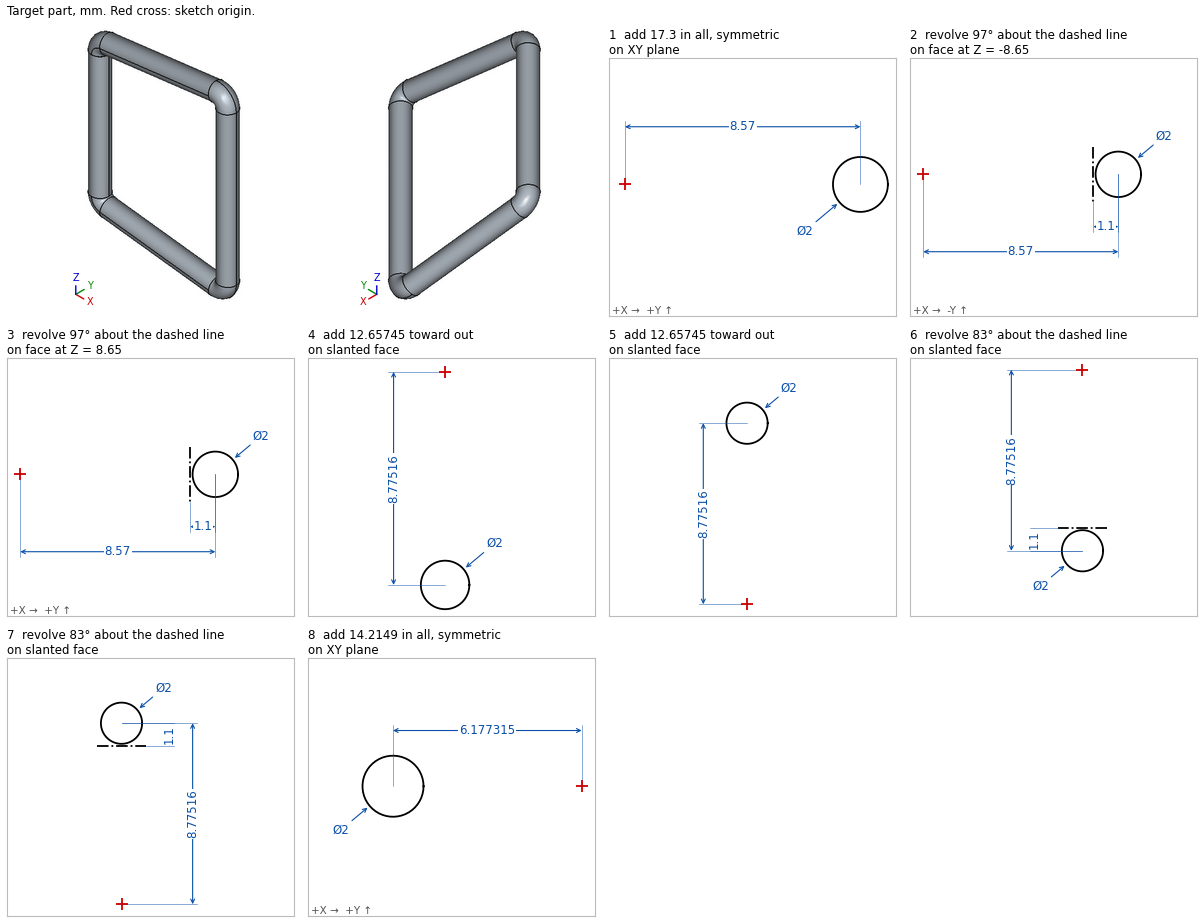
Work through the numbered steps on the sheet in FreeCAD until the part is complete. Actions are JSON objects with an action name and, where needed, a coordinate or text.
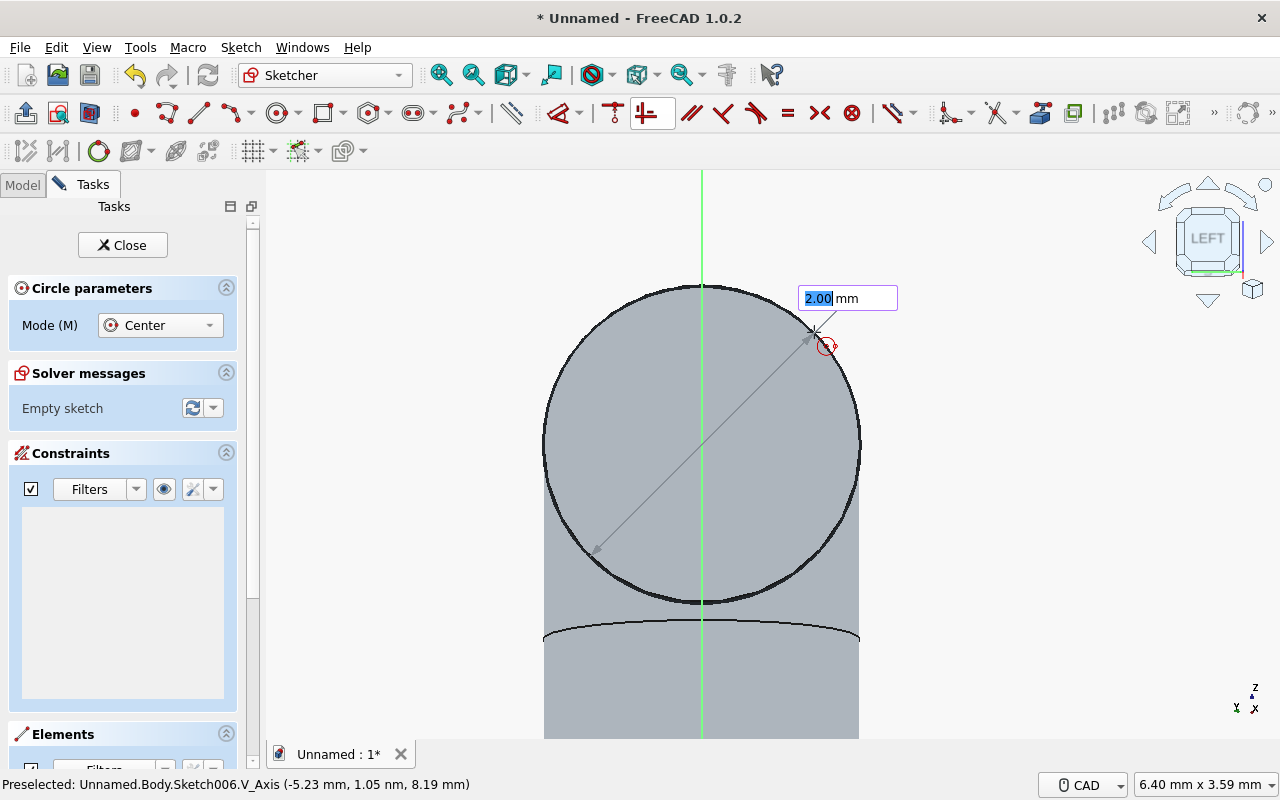
{"action": "type", "text": "2"}
{"action": "key", "text": "Return"}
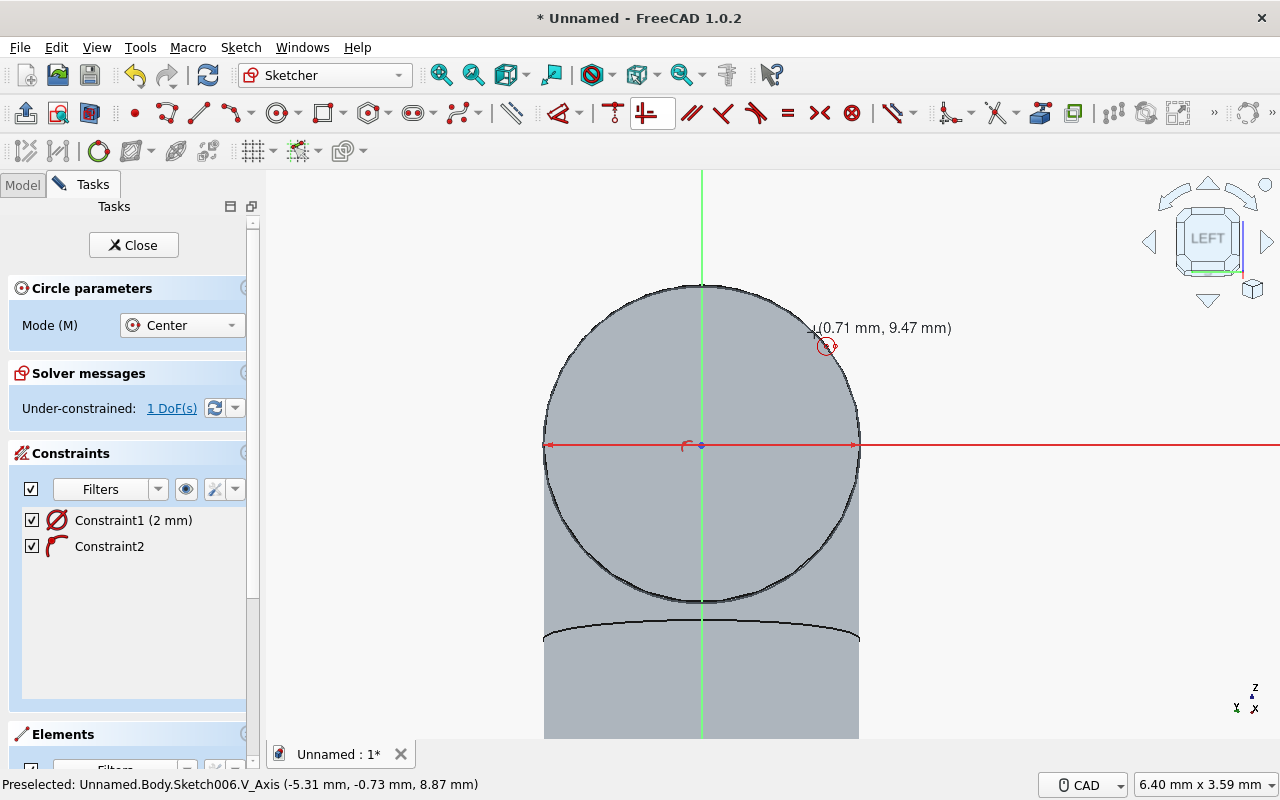
{"action": "key", "text": "g l"}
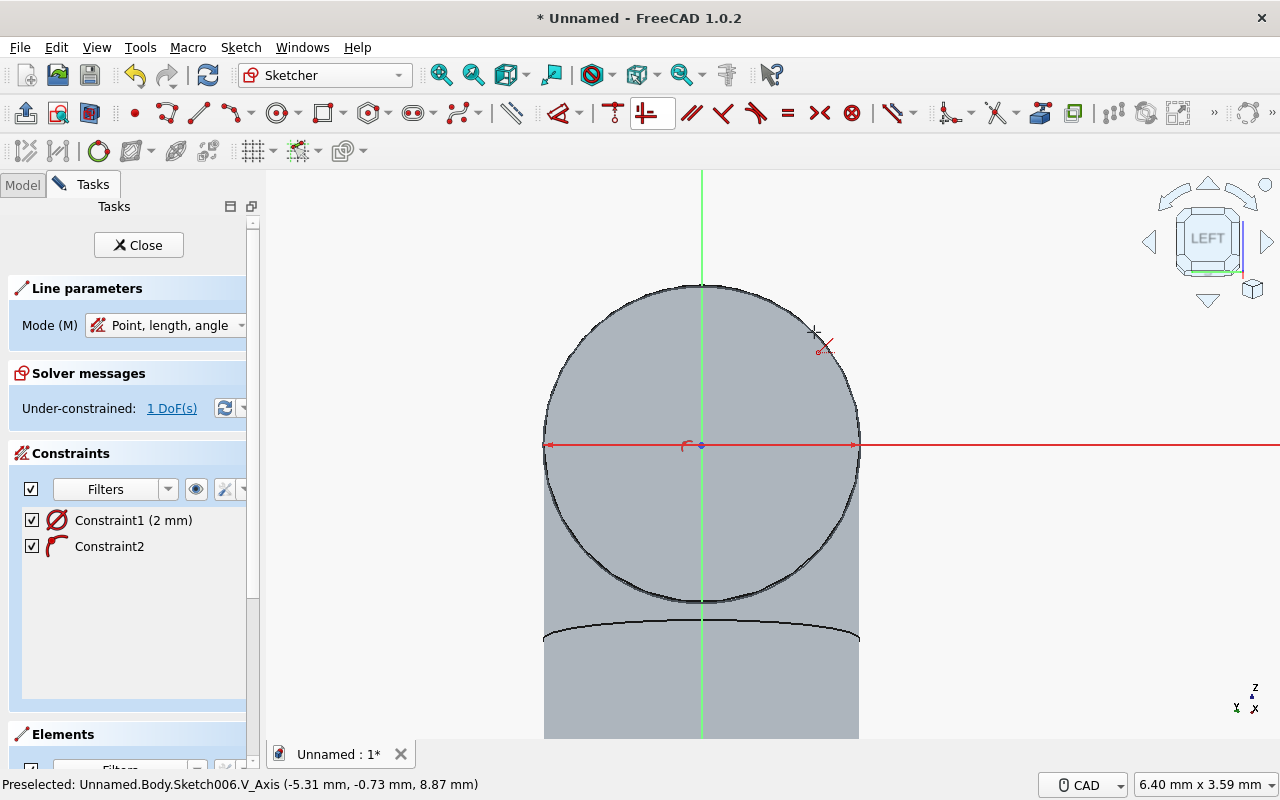
{"action": "left_click", "coordinate": [512, 618]}
{"action": "left_click", "coordinate": [892, 618]}
{"action": "key", "text": "Escape"}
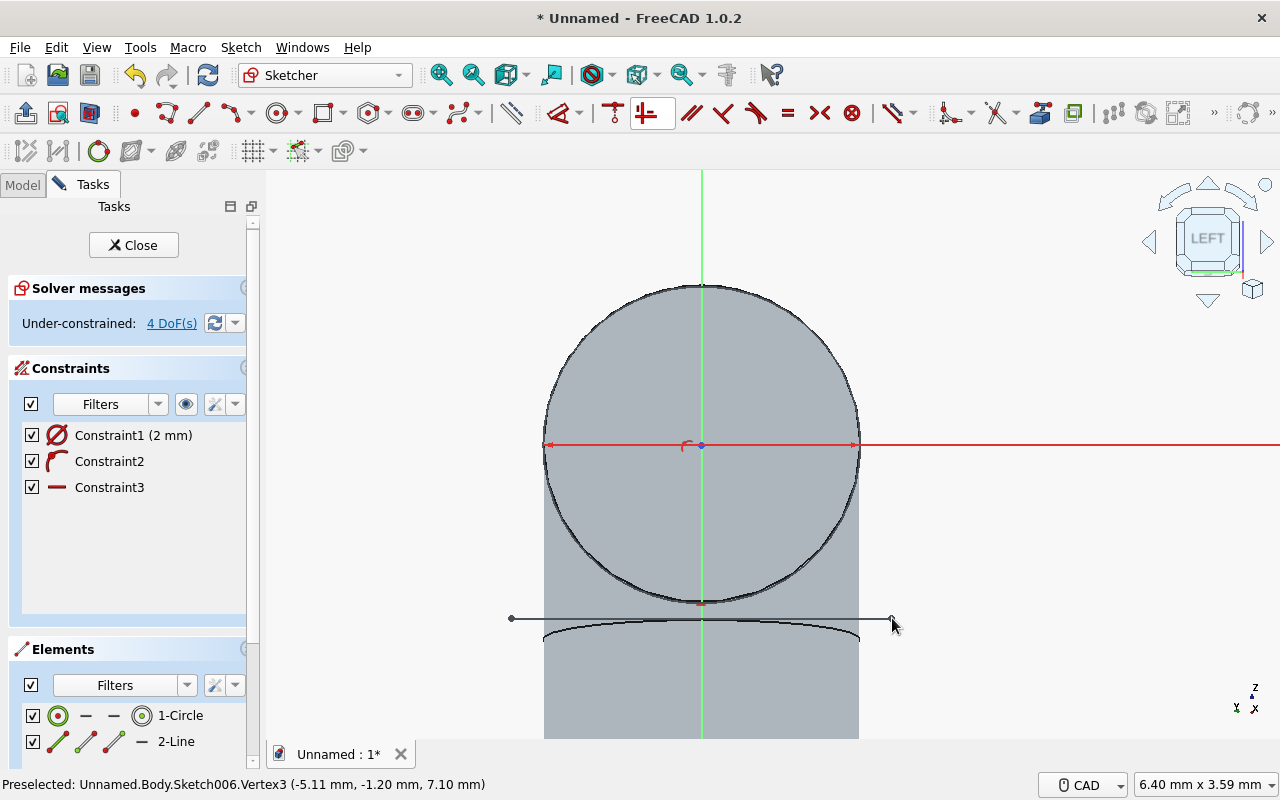
{"action": "left_click", "coordinate": [626, 619]}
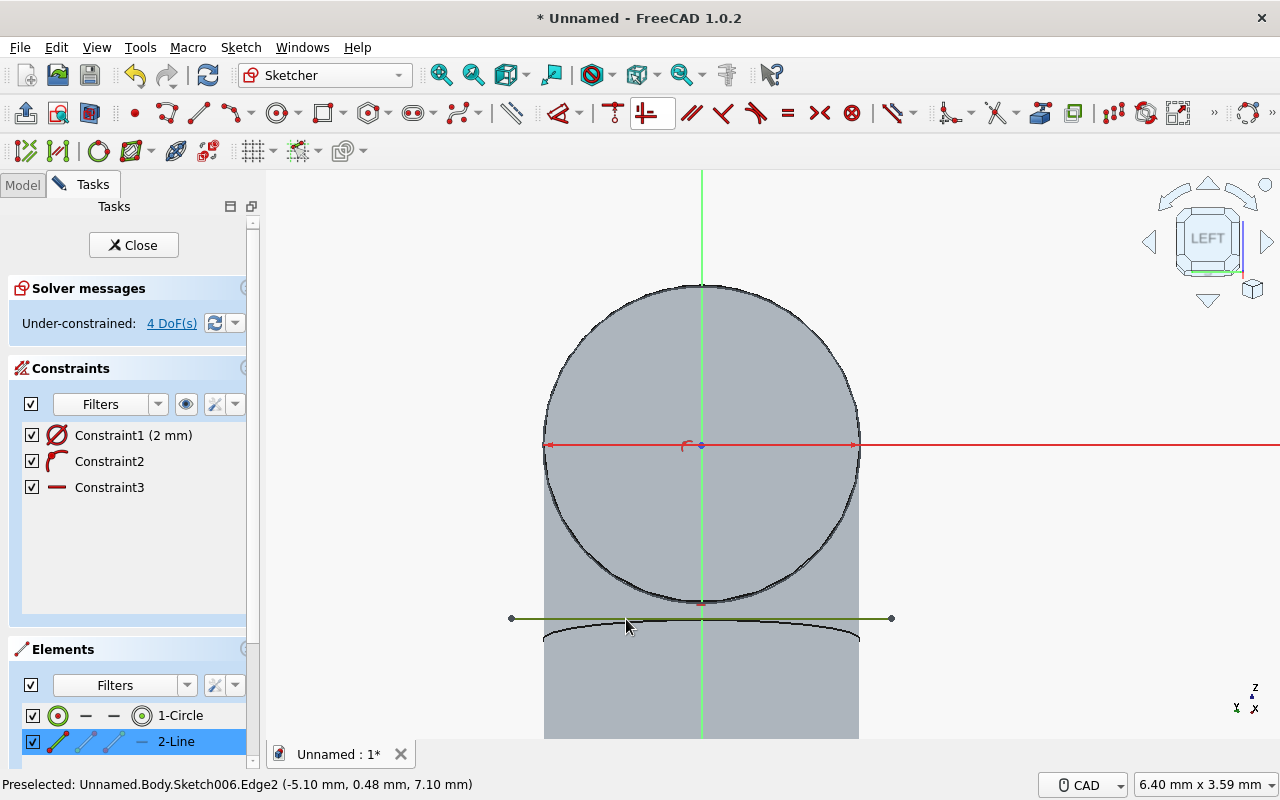
{"action": "key", "text": "g n"}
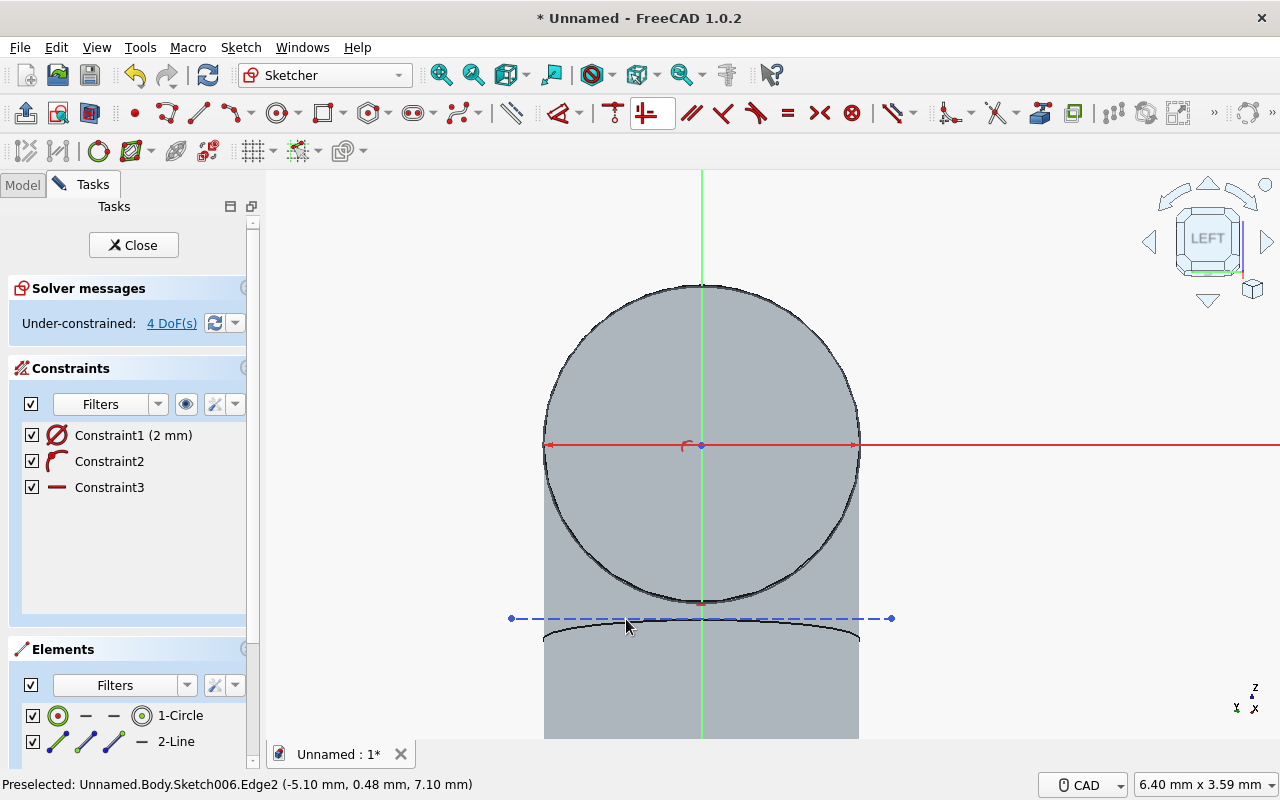
{"action": "left_click", "coordinate": [558, 114]}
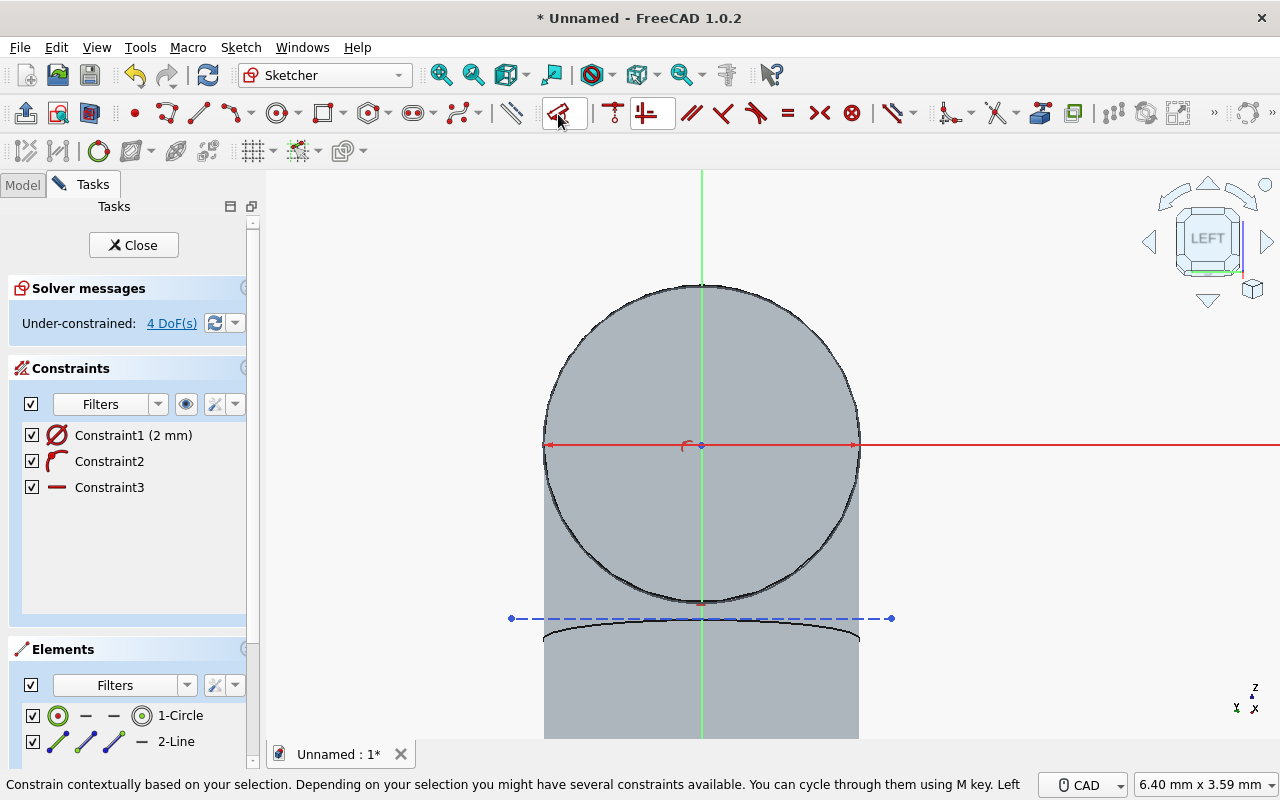
{"action": "left_click", "coordinate": [892, 619]}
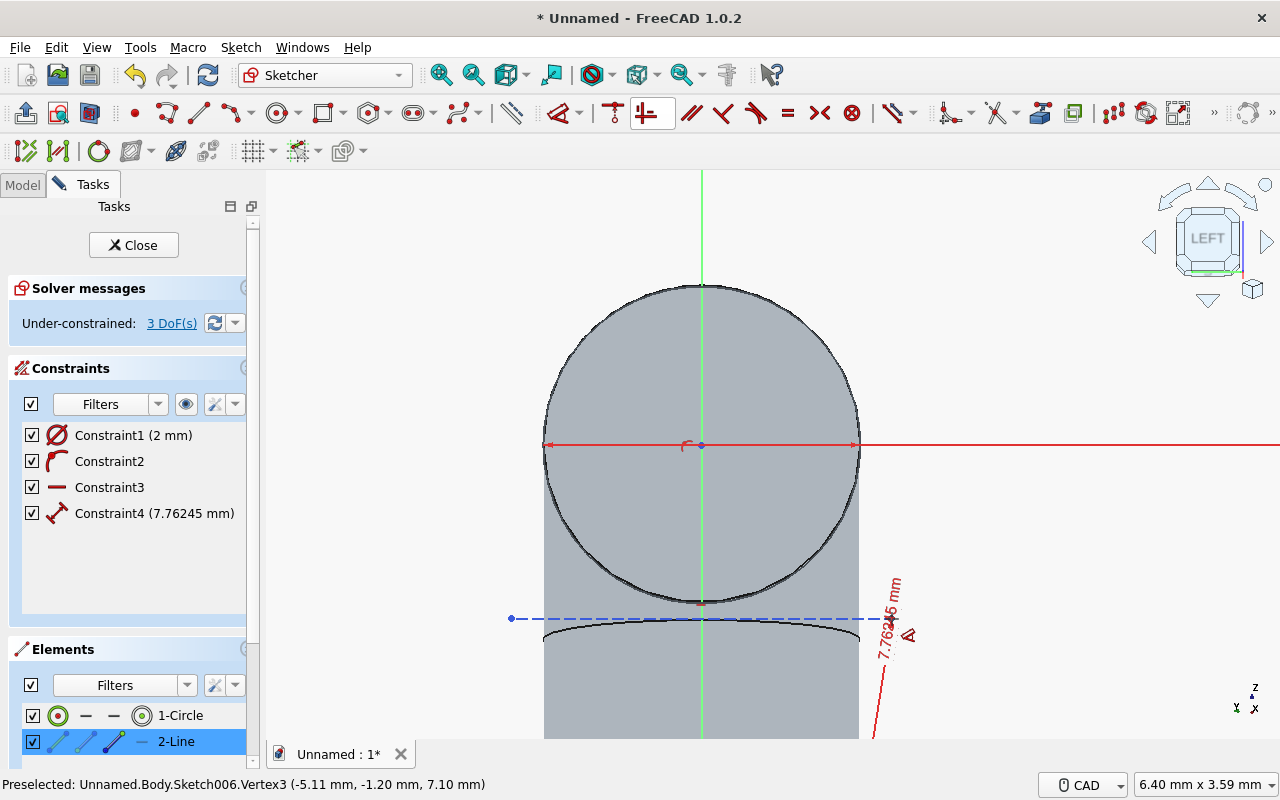
{"action": "left_click", "coordinate": [702, 445]}
{"action": "left_click", "coordinate": [926, 532]}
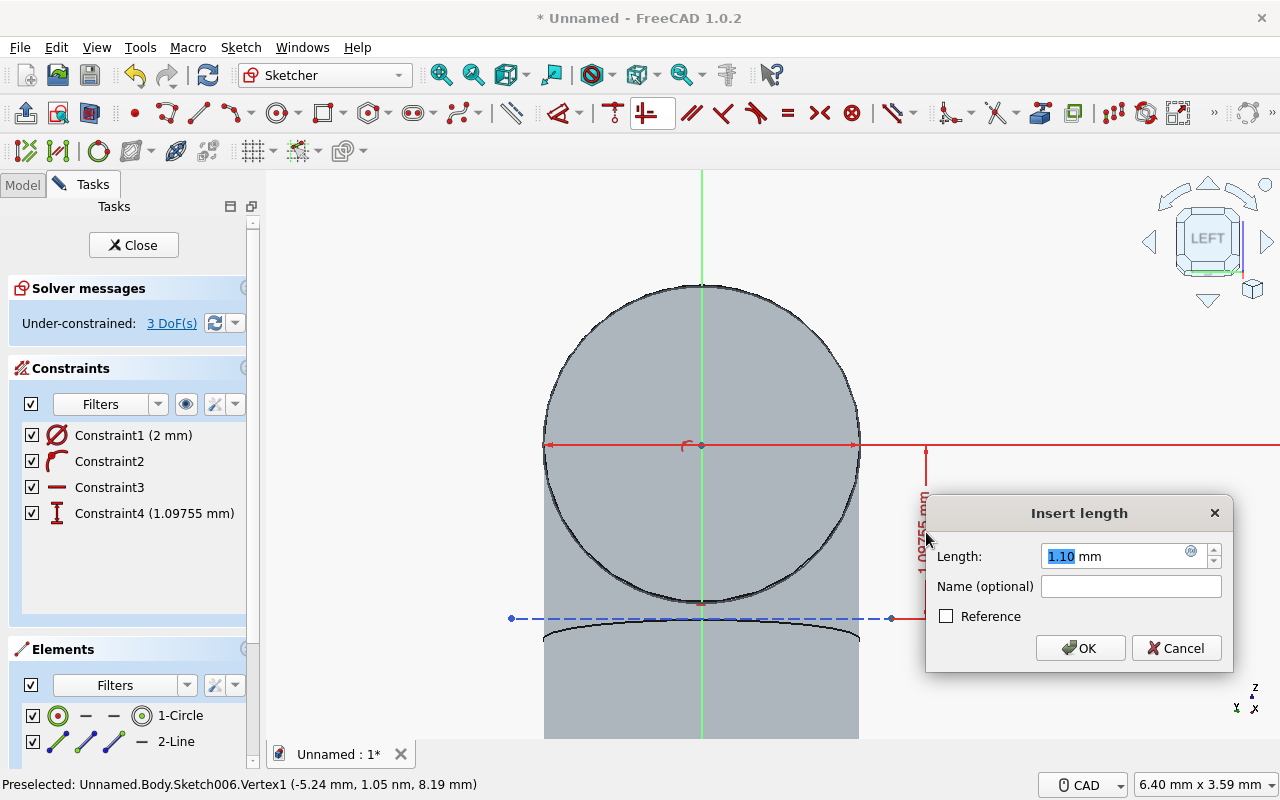
{"action": "type", "text": "1.1"}
{"action": "key", "text": "Return"}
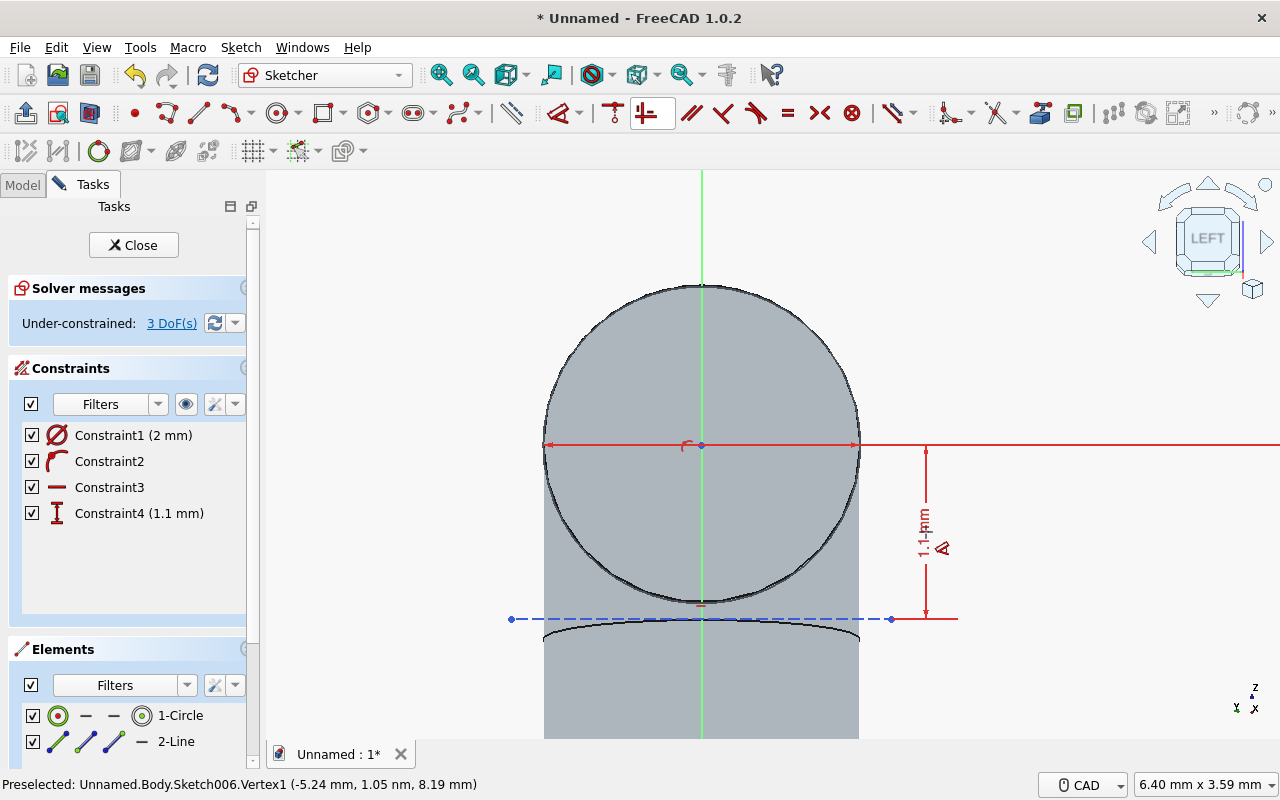
{"action": "left_click", "coordinate": [702, 445]}
{"action": "left_click", "coordinate": [736, 578]}